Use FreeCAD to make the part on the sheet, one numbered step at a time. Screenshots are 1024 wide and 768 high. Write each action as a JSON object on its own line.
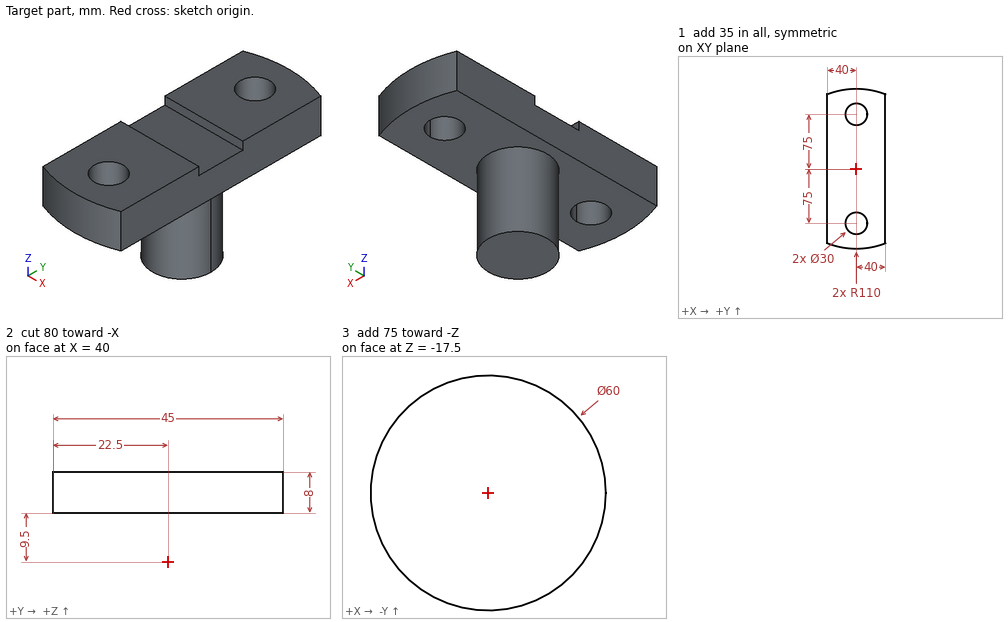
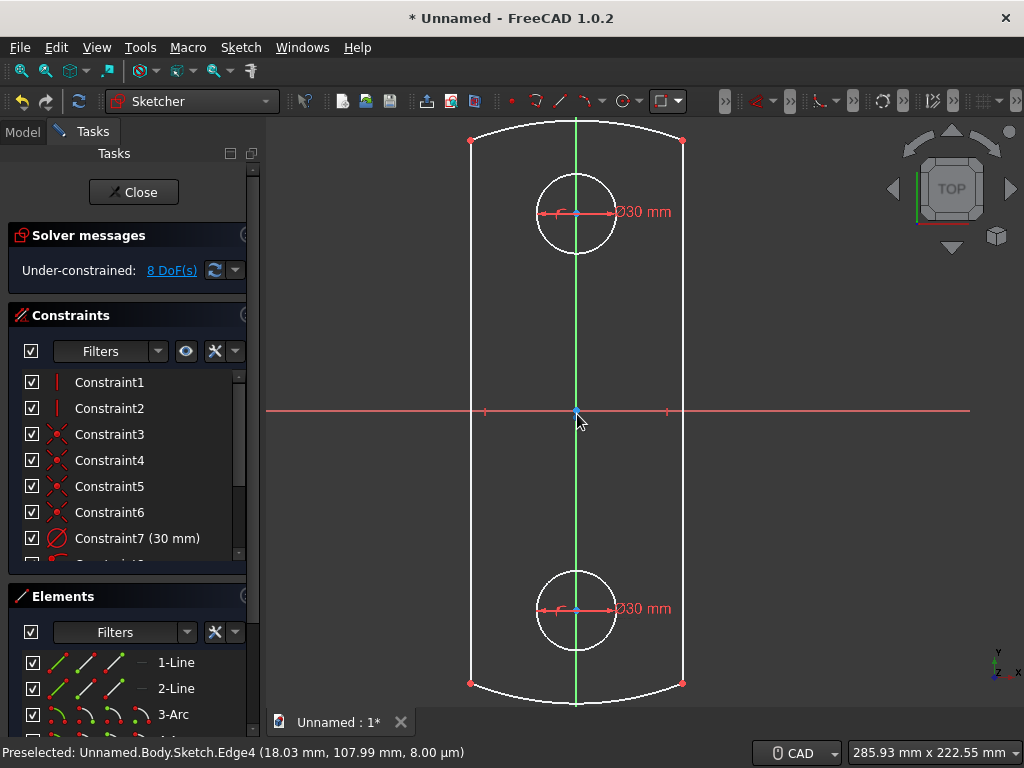
{"action": "left_click_drag", "start_coordinate": [566, 401], "coordinate": [587, 427]}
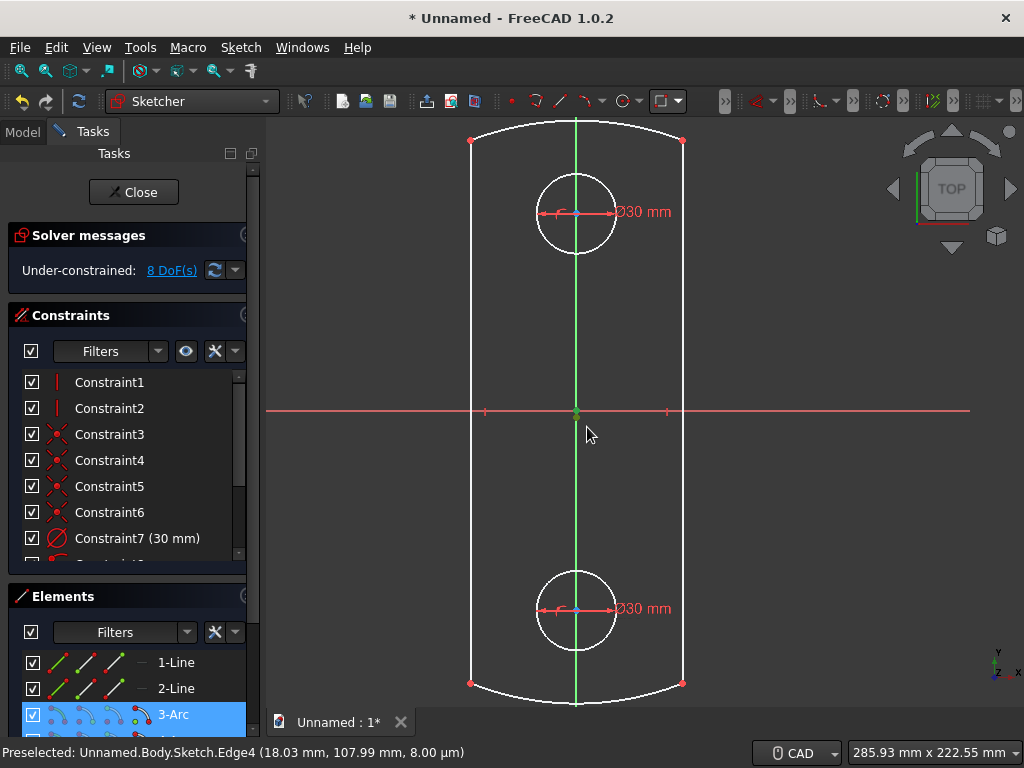
{"action": "key", "text": "c"}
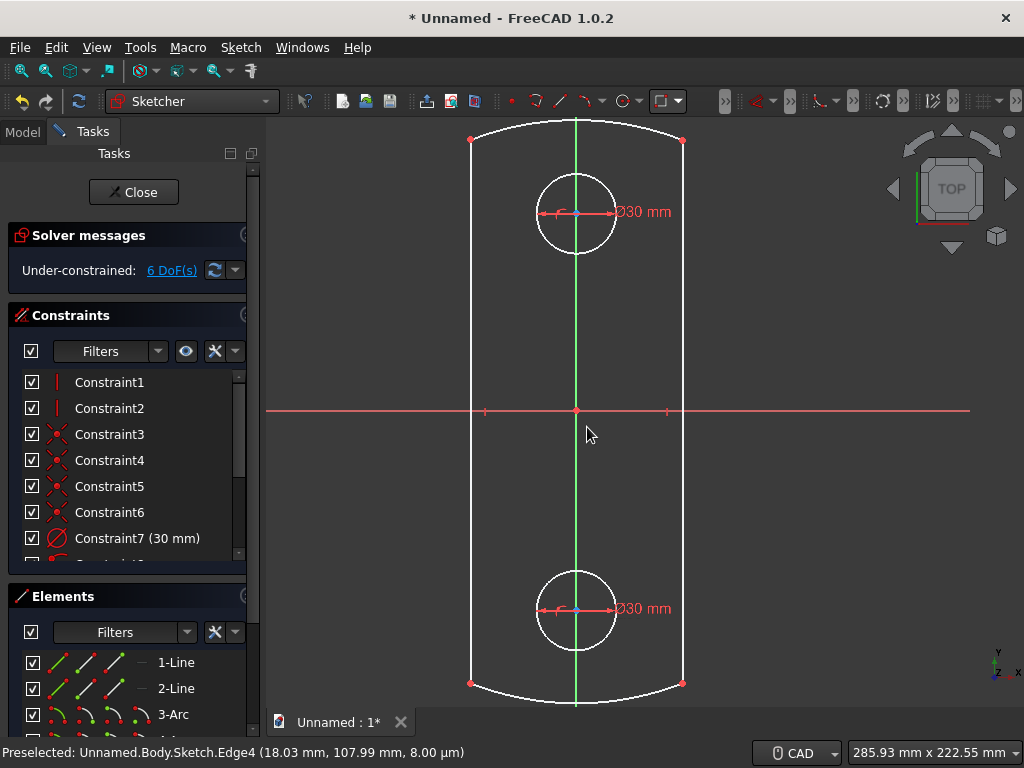
{"action": "scroll", "coordinate": [577, 414], "scroll_direction": "down", "scroll_amount": 2}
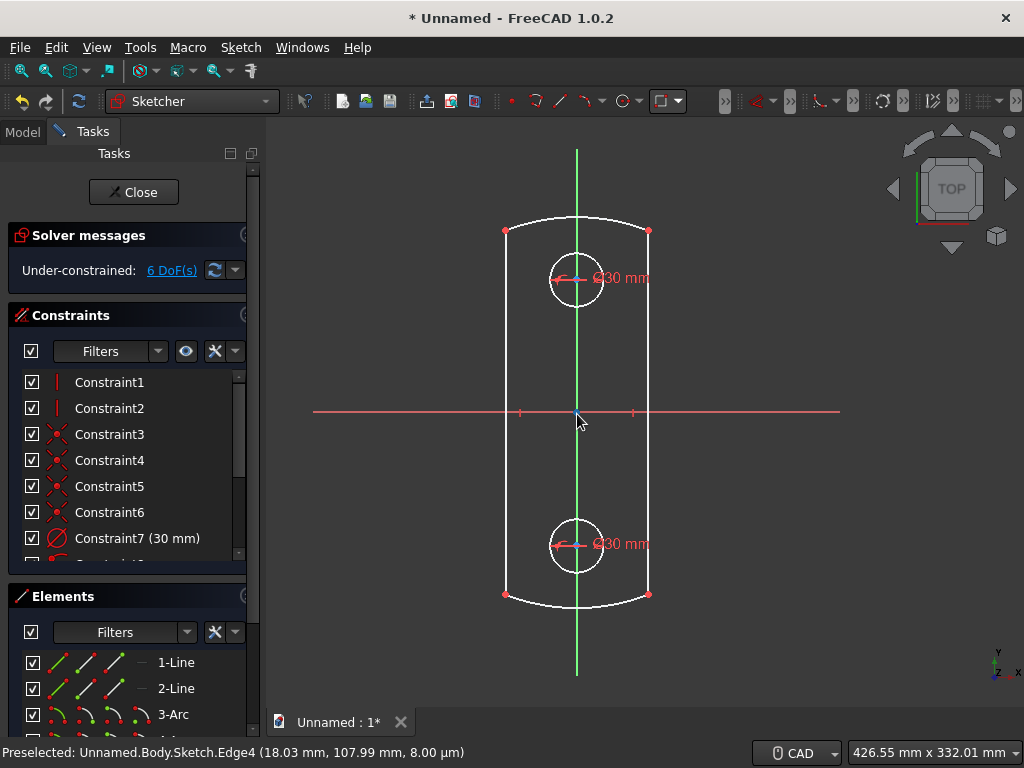
{"action": "left_click", "coordinate": [548, 606]}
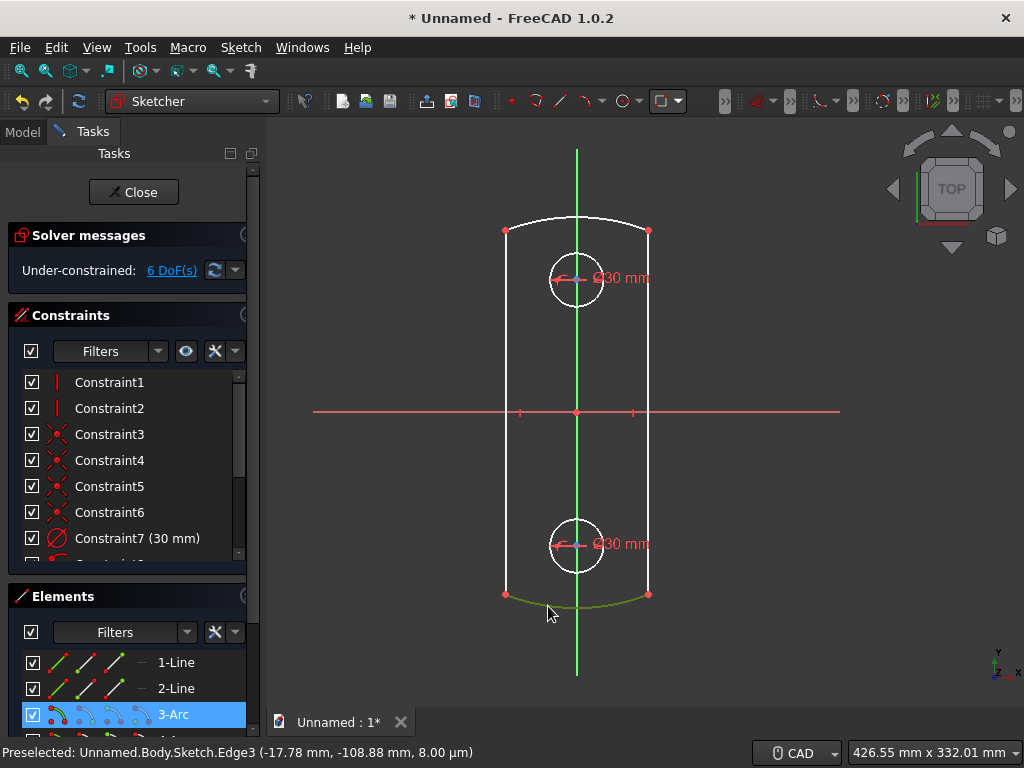
{"action": "left_click", "coordinate": [606, 219]}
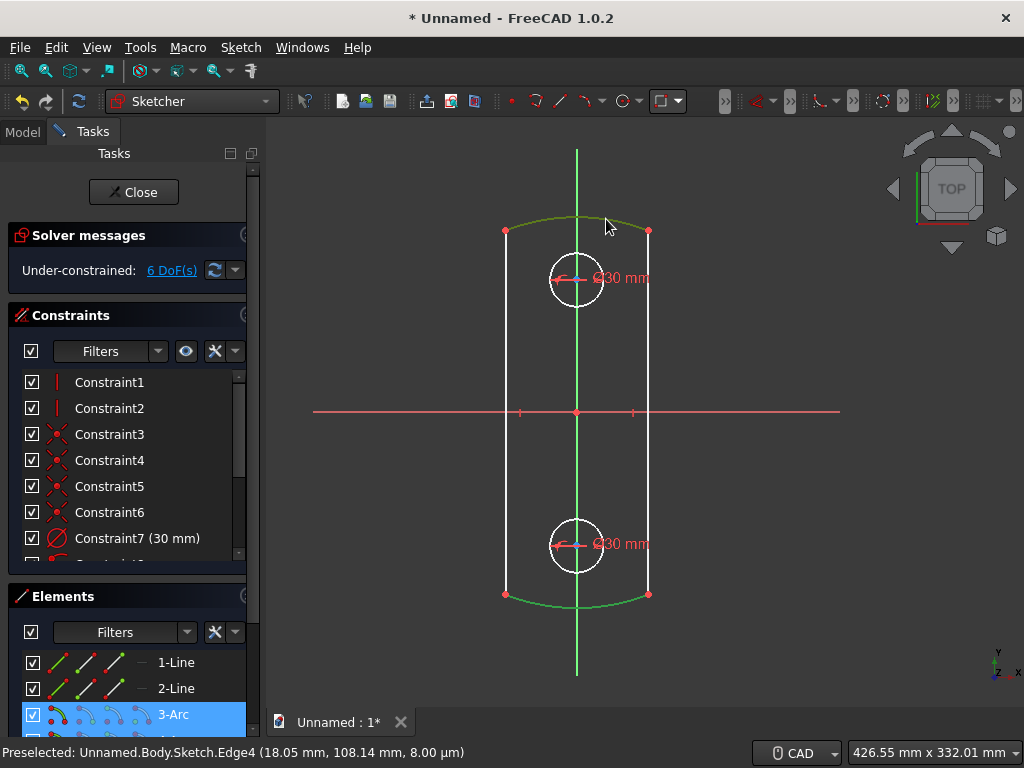
{"action": "key", "text": "e"}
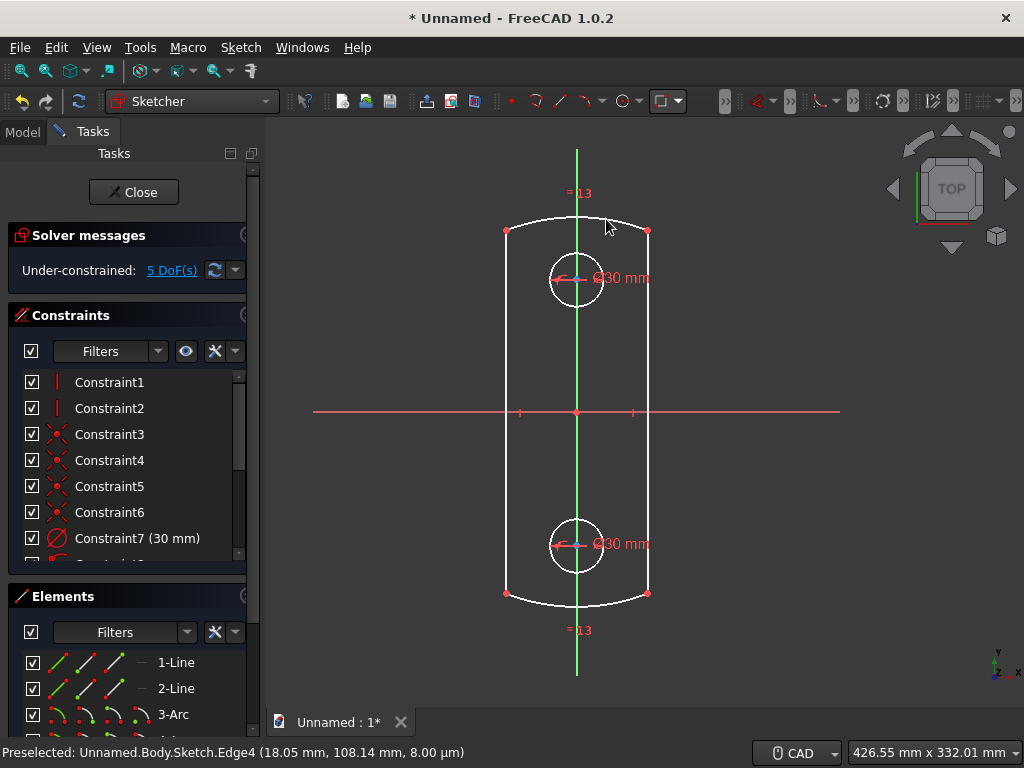
{"action": "key", "text": "d"}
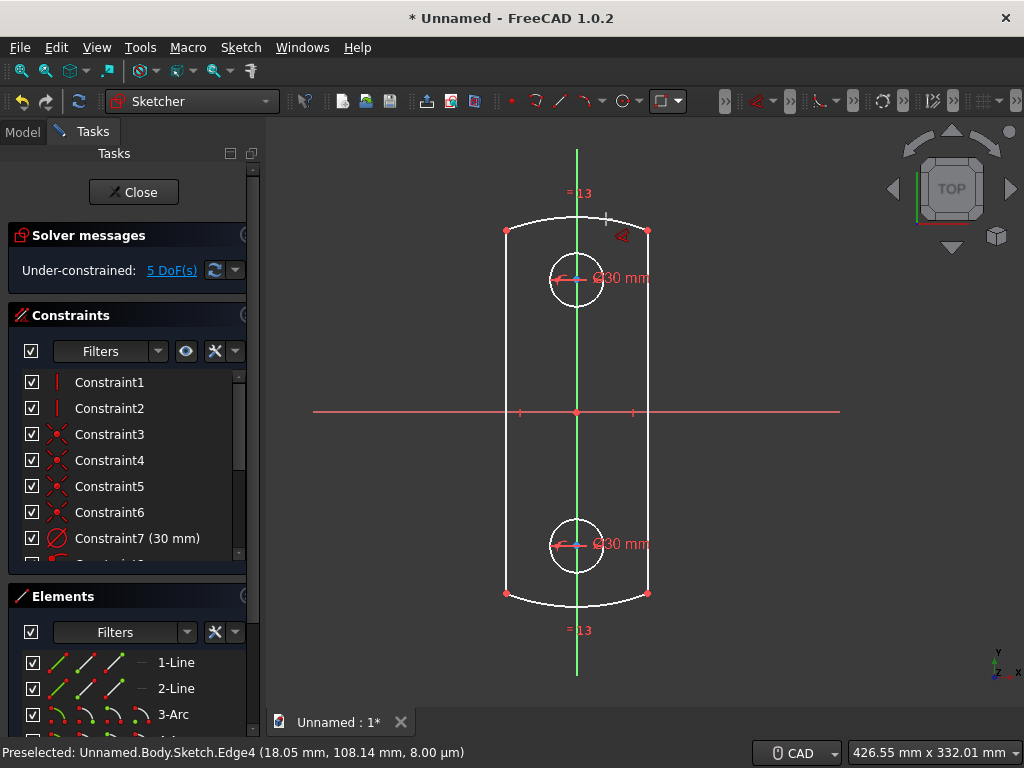
{"action": "left_click", "coordinate": [548, 605]}
{"action": "left_click", "coordinate": [543, 637]}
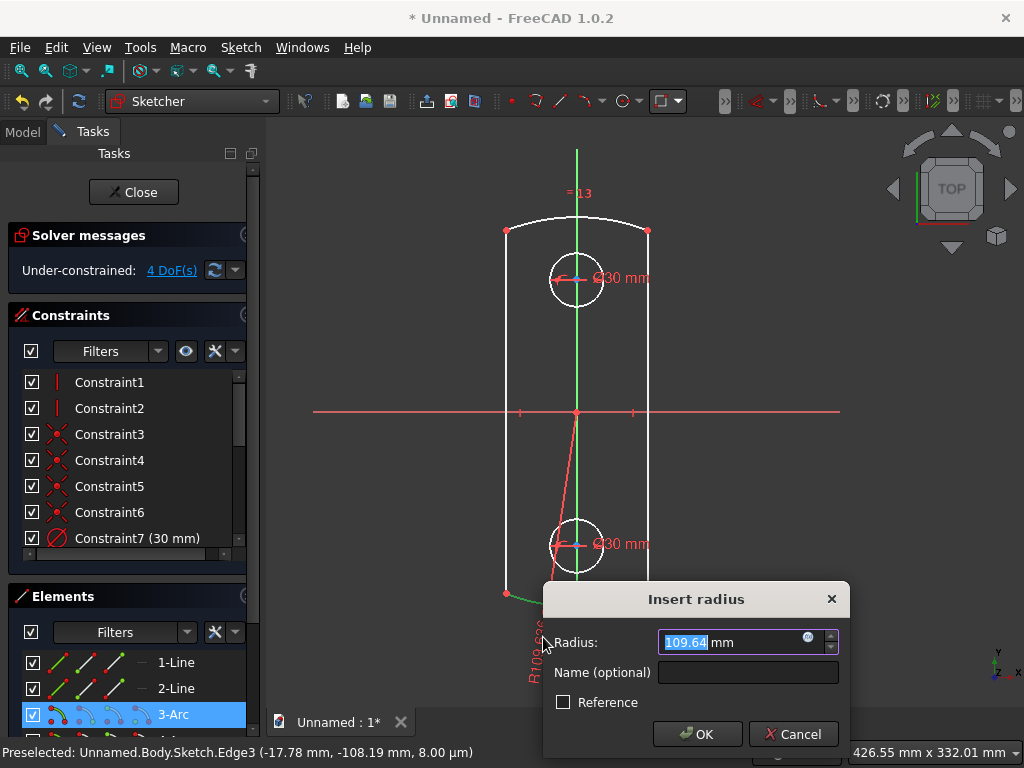
{"action": "type", "text": "110"}
{"action": "key", "text": "Return"}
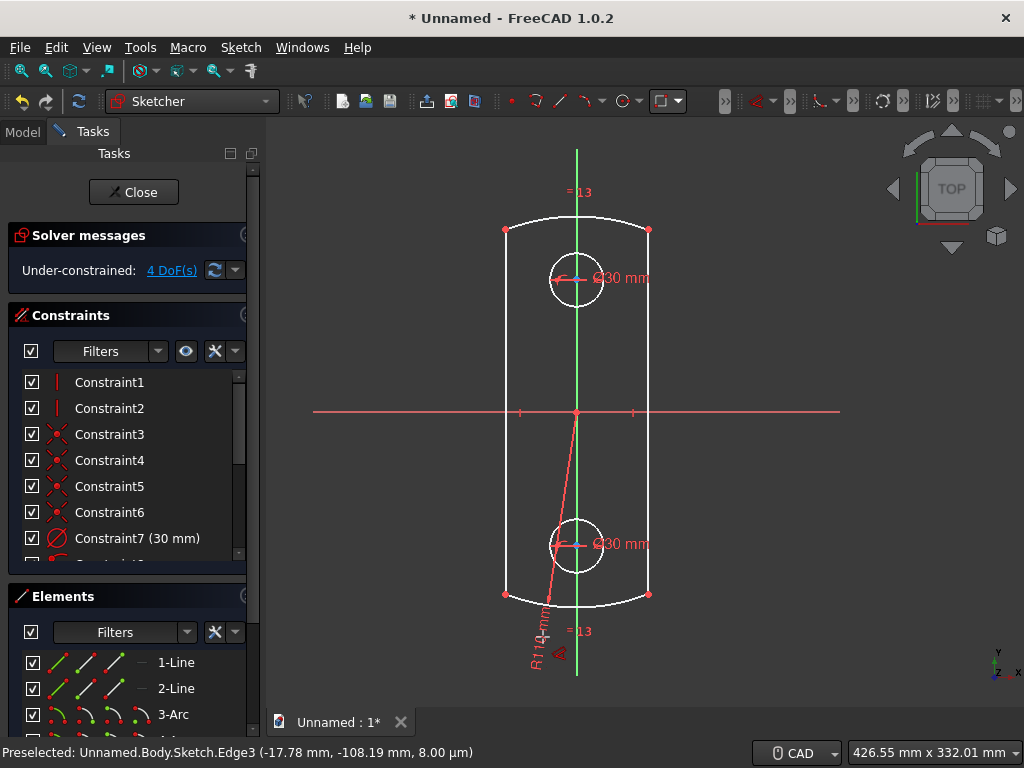
{"action": "left_click", "coordinate": [577, 546]}
{"action": "left_click", "coordinate": [611, 479]}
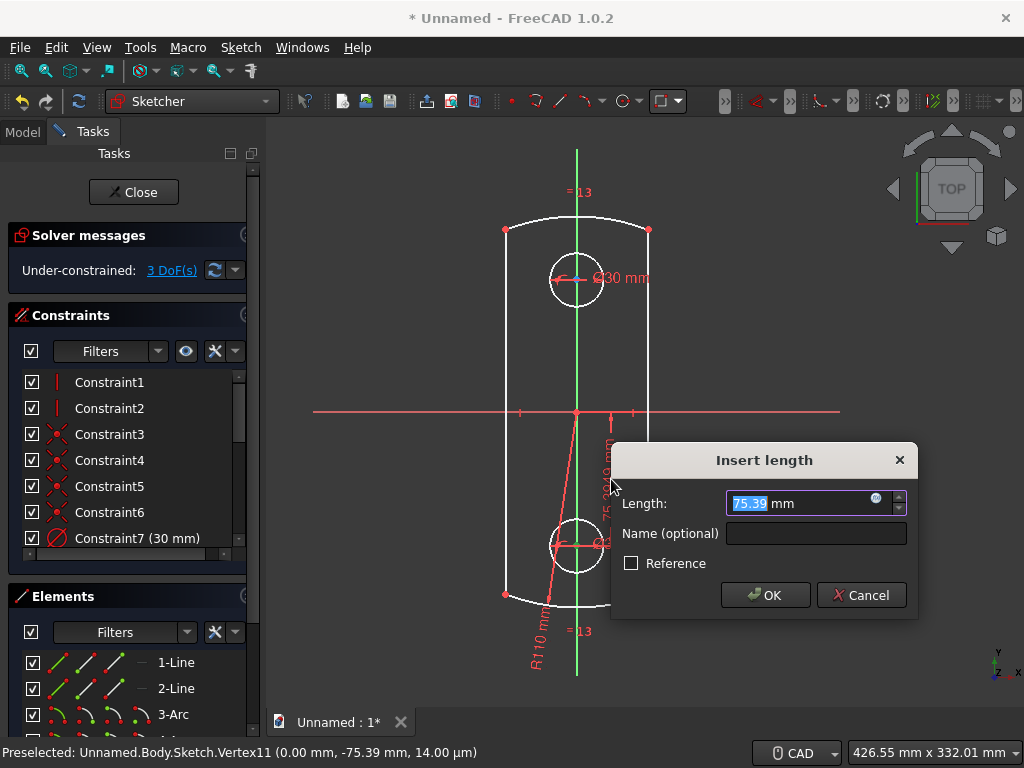
{"action": "type", "text": "75"}
{"action": "key", "text": "Return"}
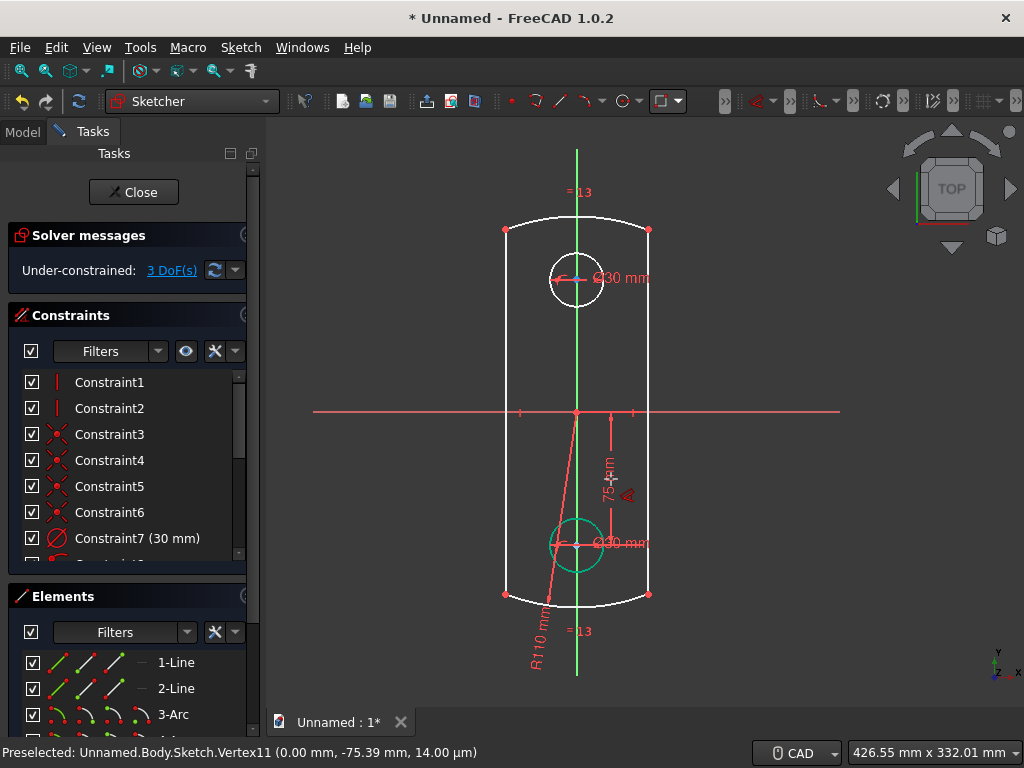
{"action": "left_click", "coordinate": [577, 280]}
{"action": "left_click", "coordinate": [611, 346]}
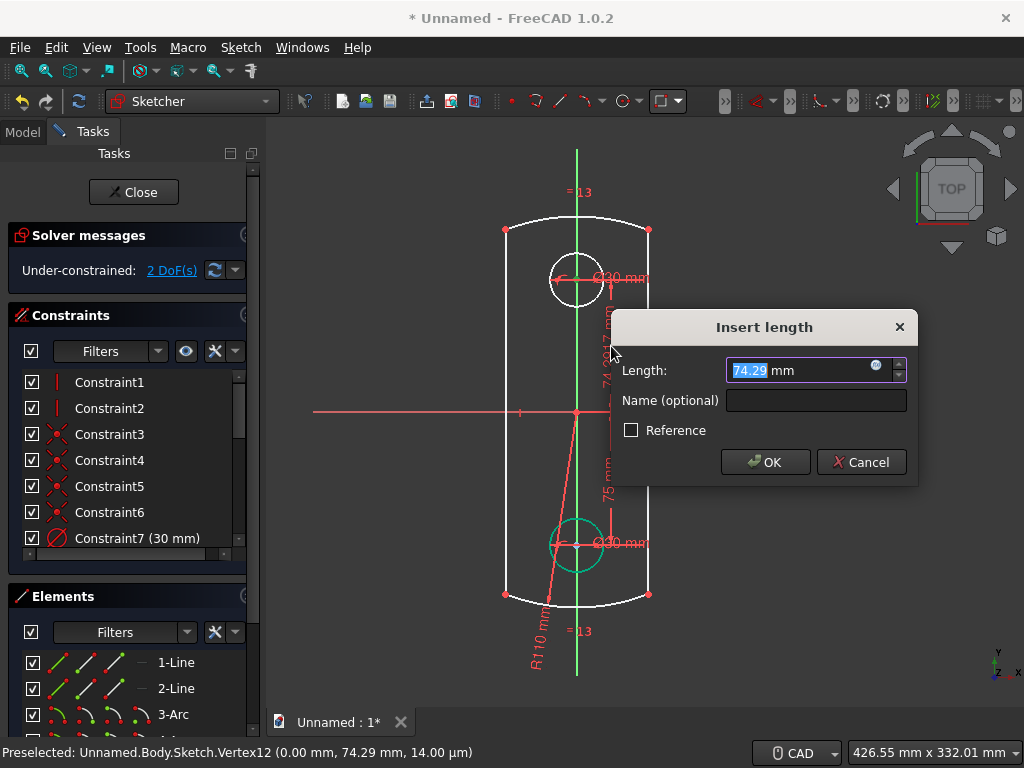
{"action": "type", "text": "75"}
{"action": "key", "text": "Return"}